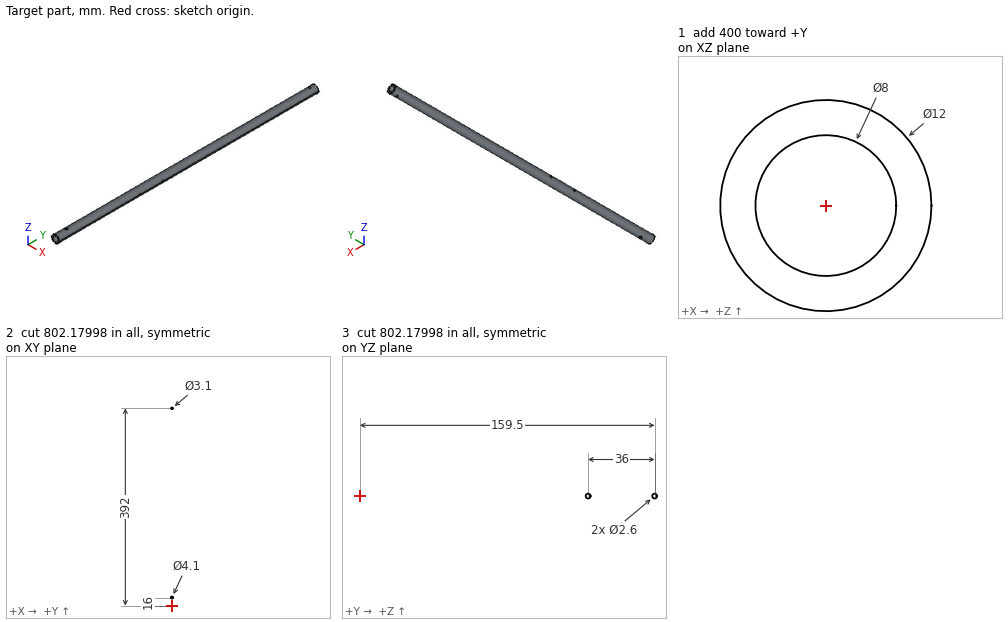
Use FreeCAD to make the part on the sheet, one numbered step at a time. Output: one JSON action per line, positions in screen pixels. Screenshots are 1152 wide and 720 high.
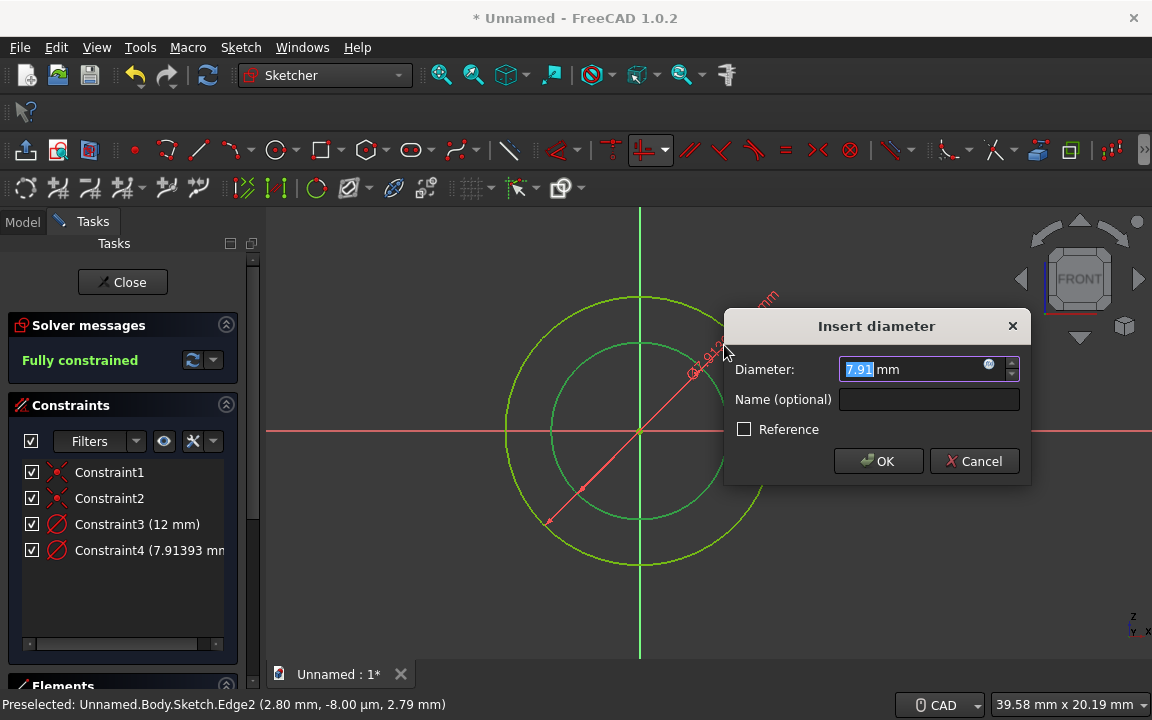
{"action": "type", "text": "8"}
{"action": "key", "text": "Return"}
{"action": "key", "text": "Escape"}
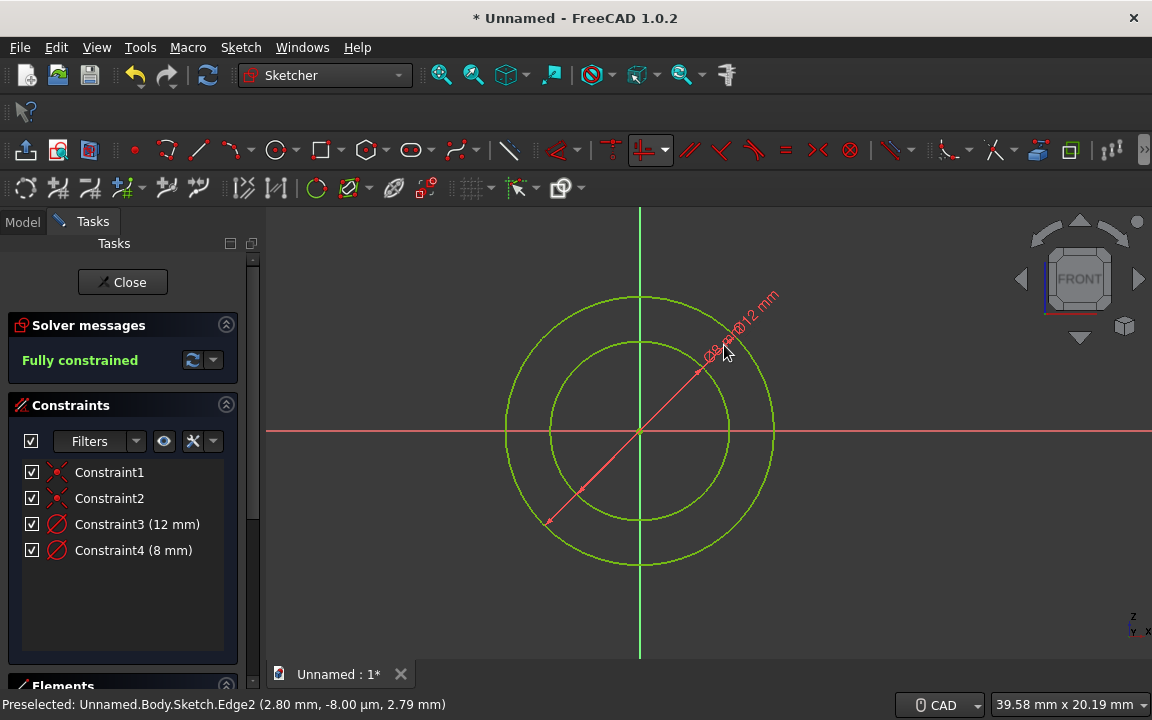
{"action": "left_click", "coordinate": [123, 282]}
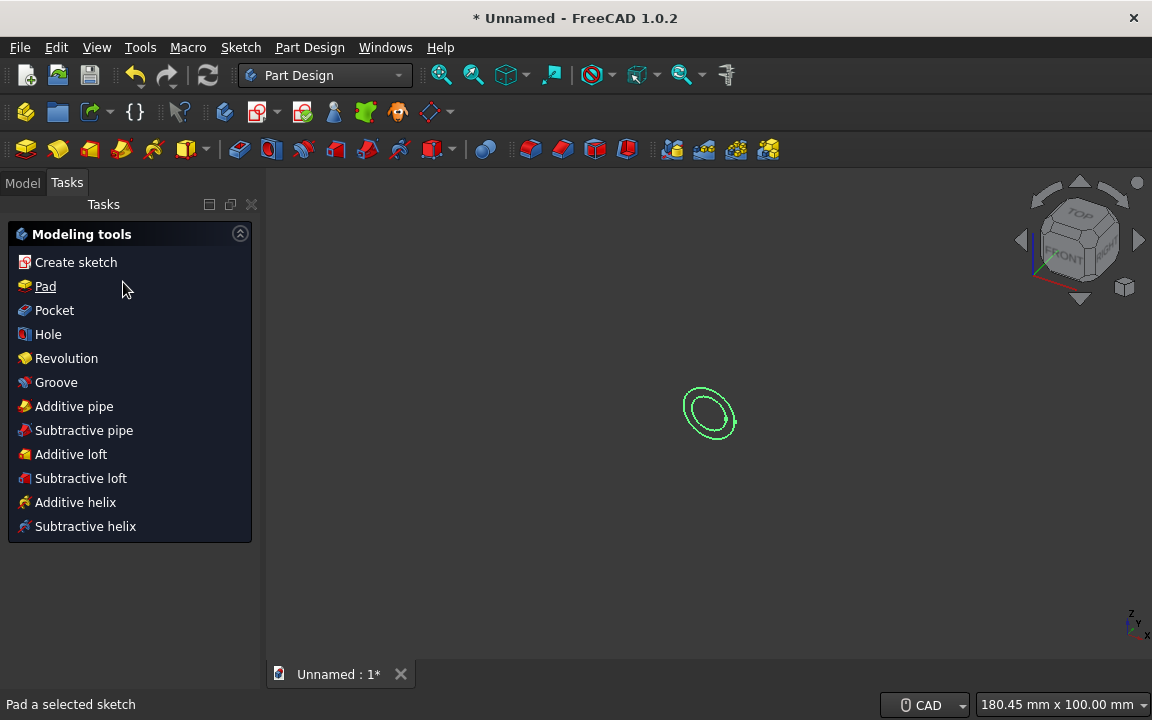
{"action": "left_click", "coordinate": [26, 150]}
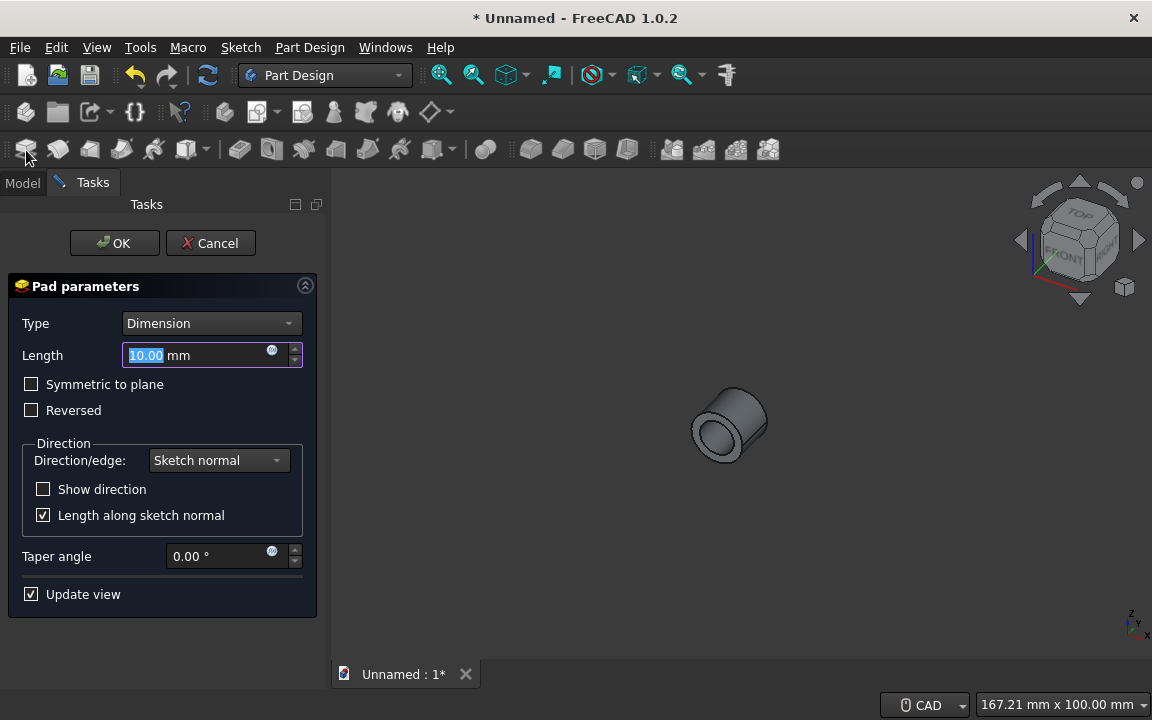
{"action": "type", "text": "400"}
{"action": "key", "text": "Tab"}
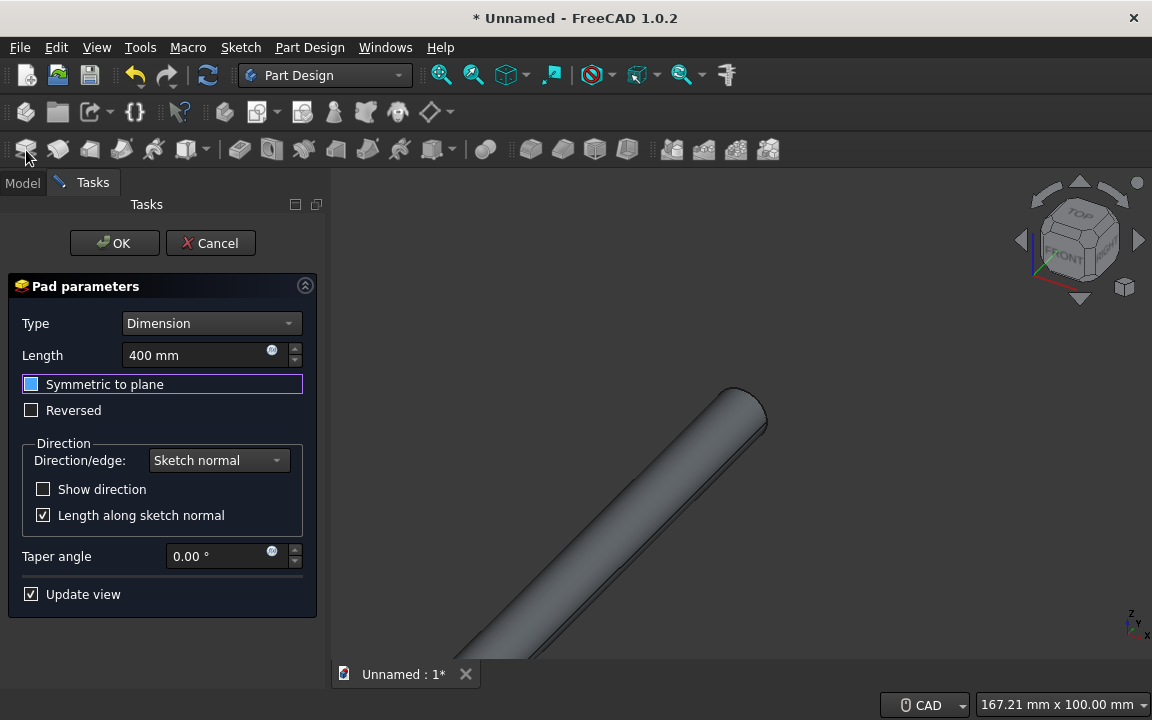
{"action": "left_click", "coordinate": [30, 410]}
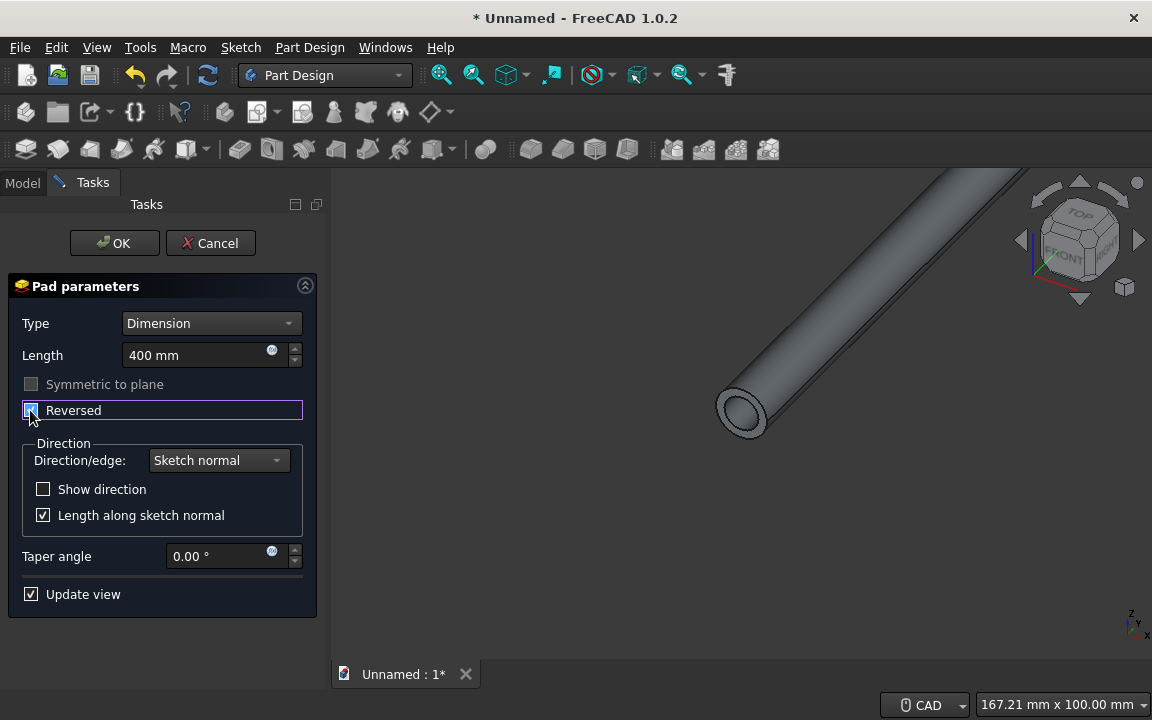
{"action": "left_click", "coordinate": [115, 243]}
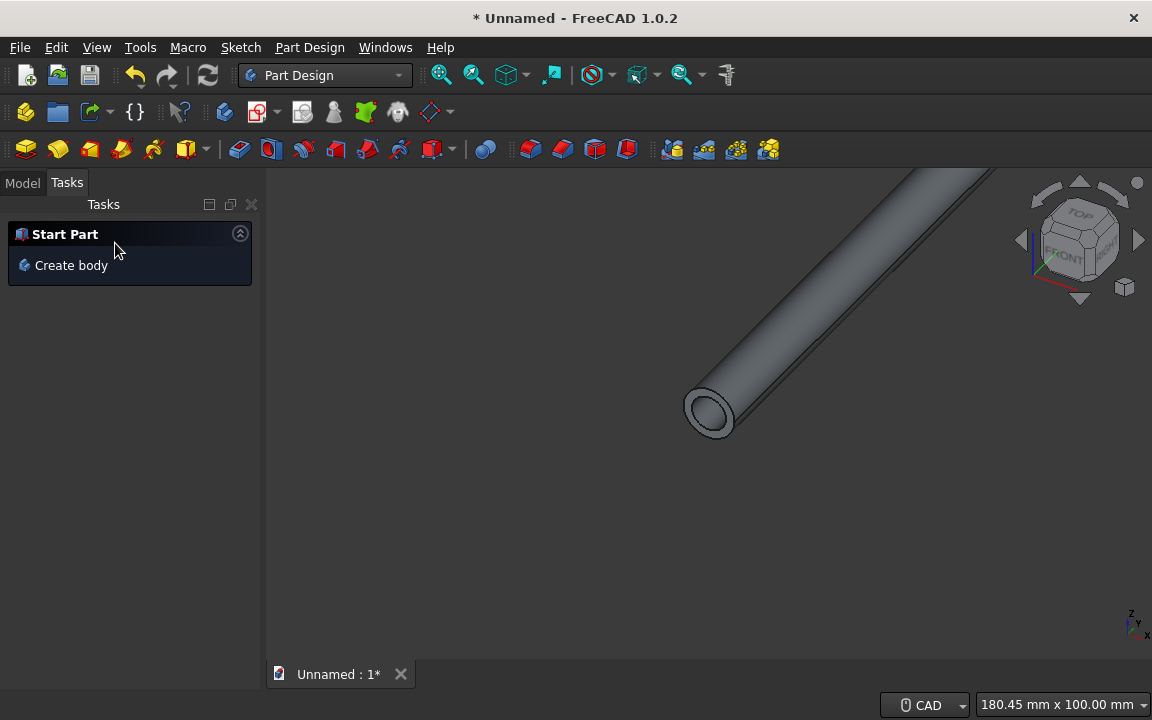
{"action": "left_click", "coordinate": [442, 76]}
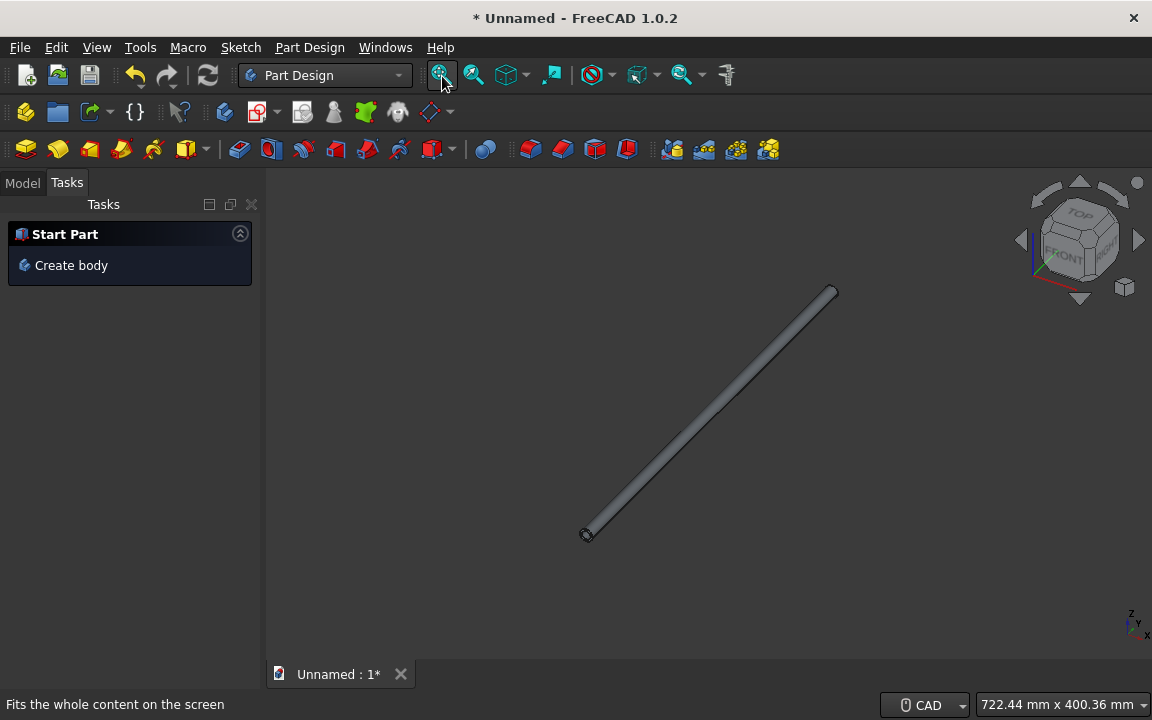
{"action": "left_click", "coordinate": [258, 112]}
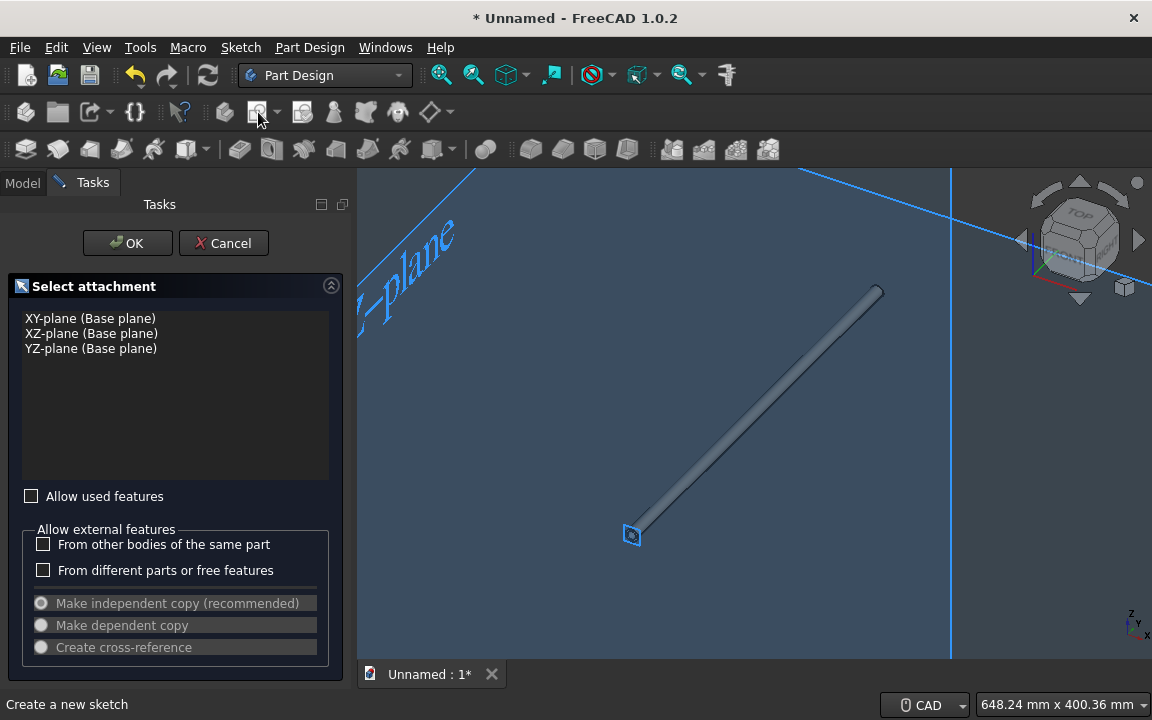
{"action": "left_click", "coordinate": [82, 318]}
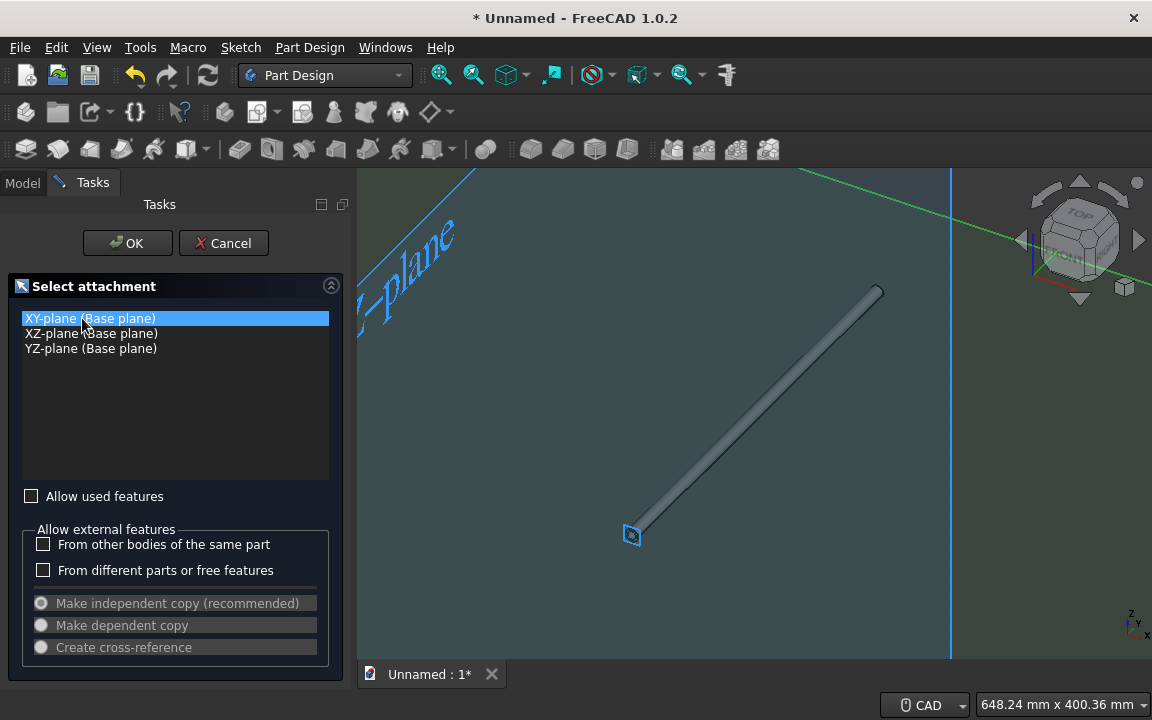
{"action": "left_click", "coordinate": [128, 243]}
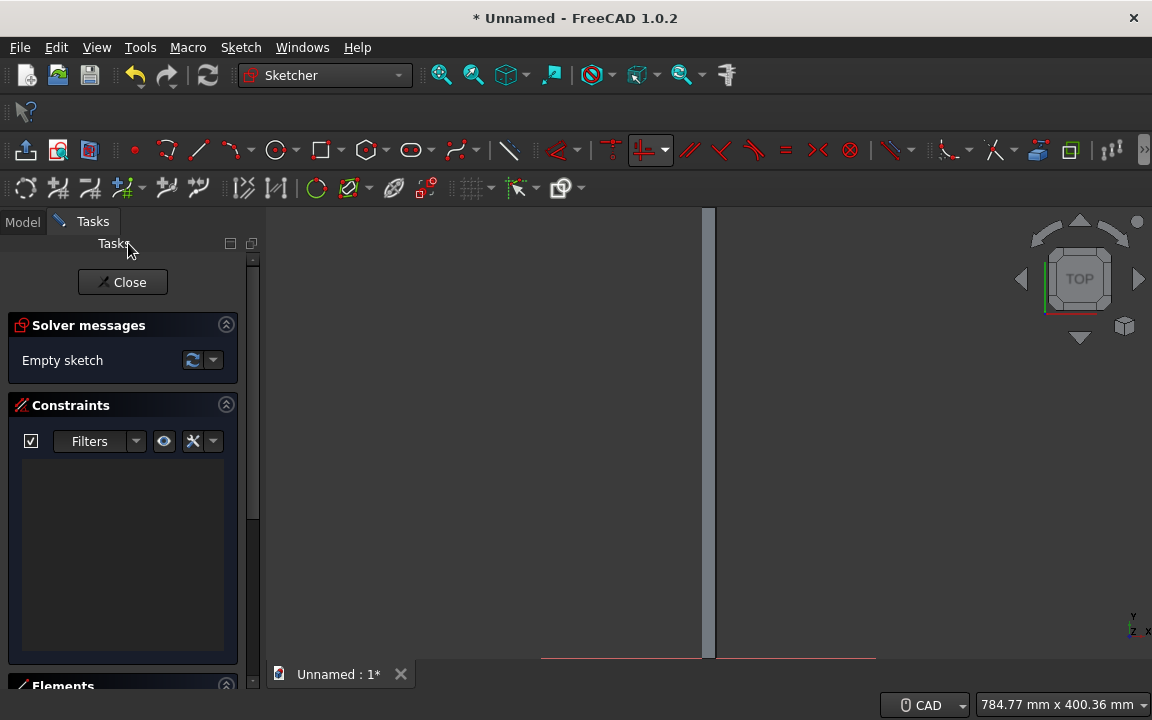
{"action": "key", "text": "q s"}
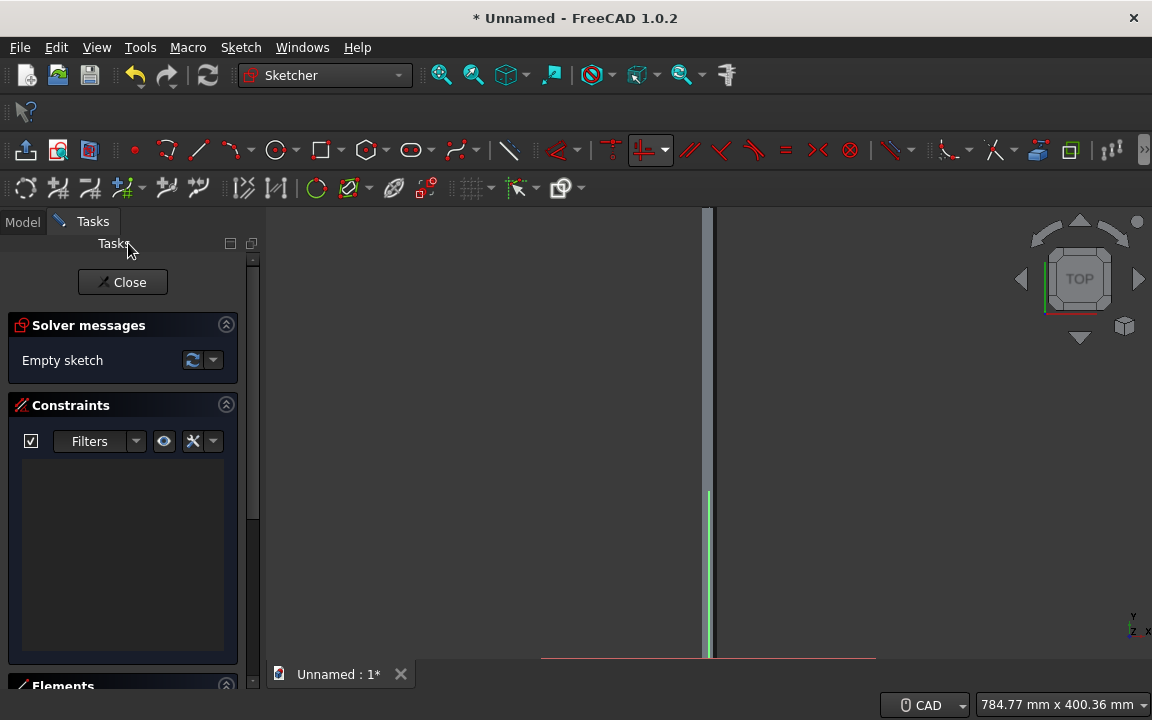
{"action": "scroll", "coordinate": [501, 426], "scroll_direction": "down", "scroll_amount": 2}